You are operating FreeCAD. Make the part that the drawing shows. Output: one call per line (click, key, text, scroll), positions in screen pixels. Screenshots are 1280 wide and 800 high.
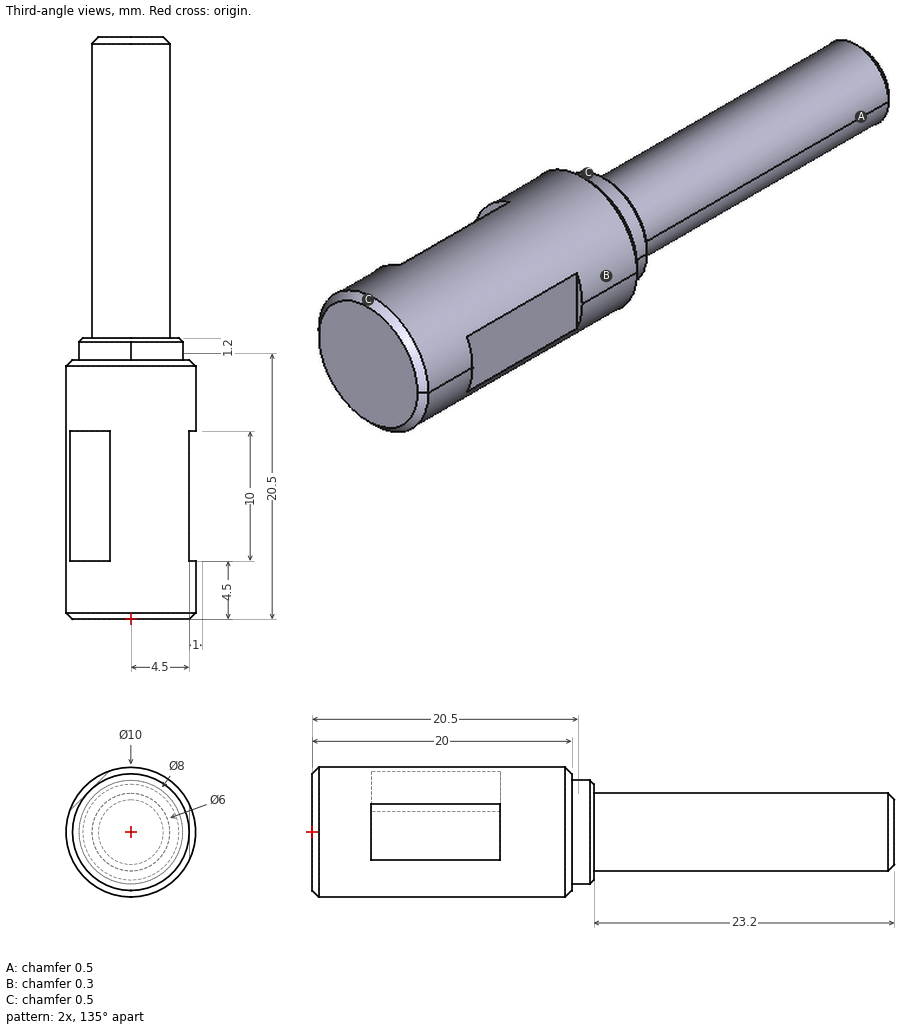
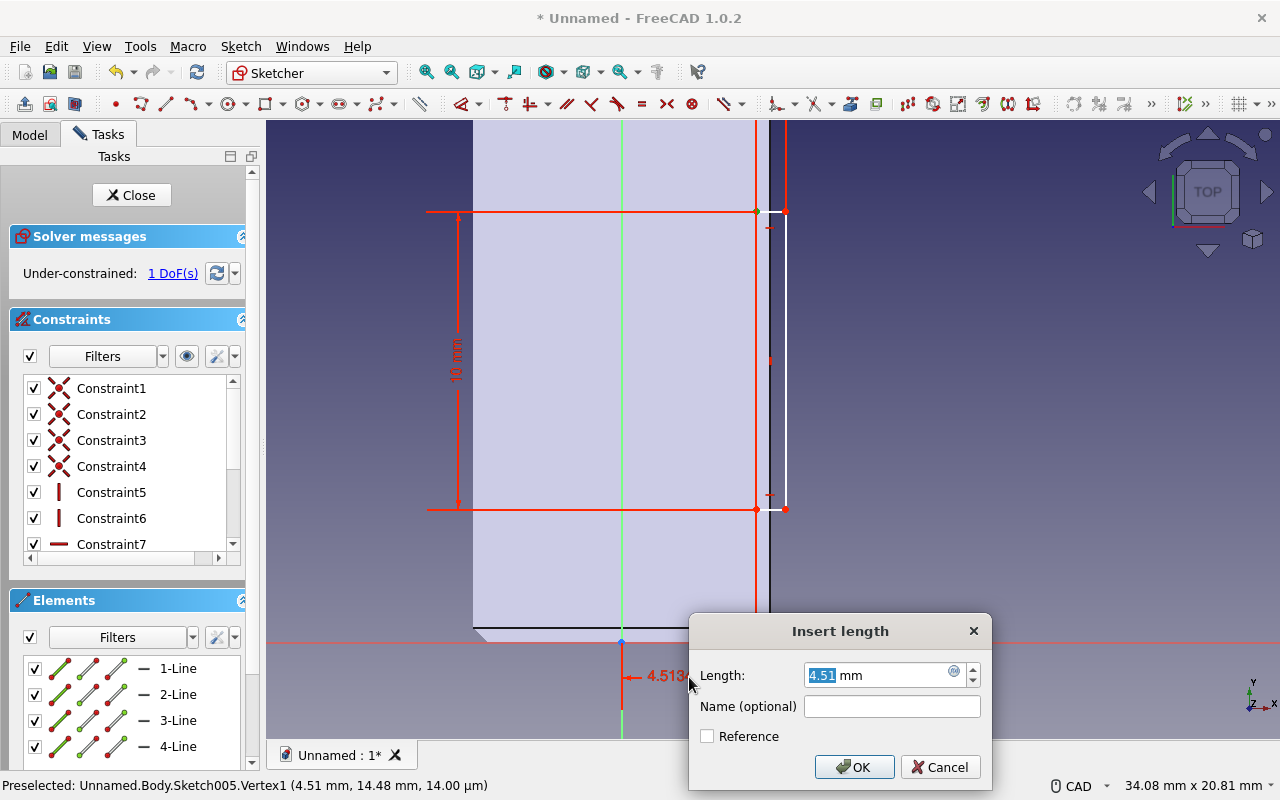
text(4.5)
key(Return)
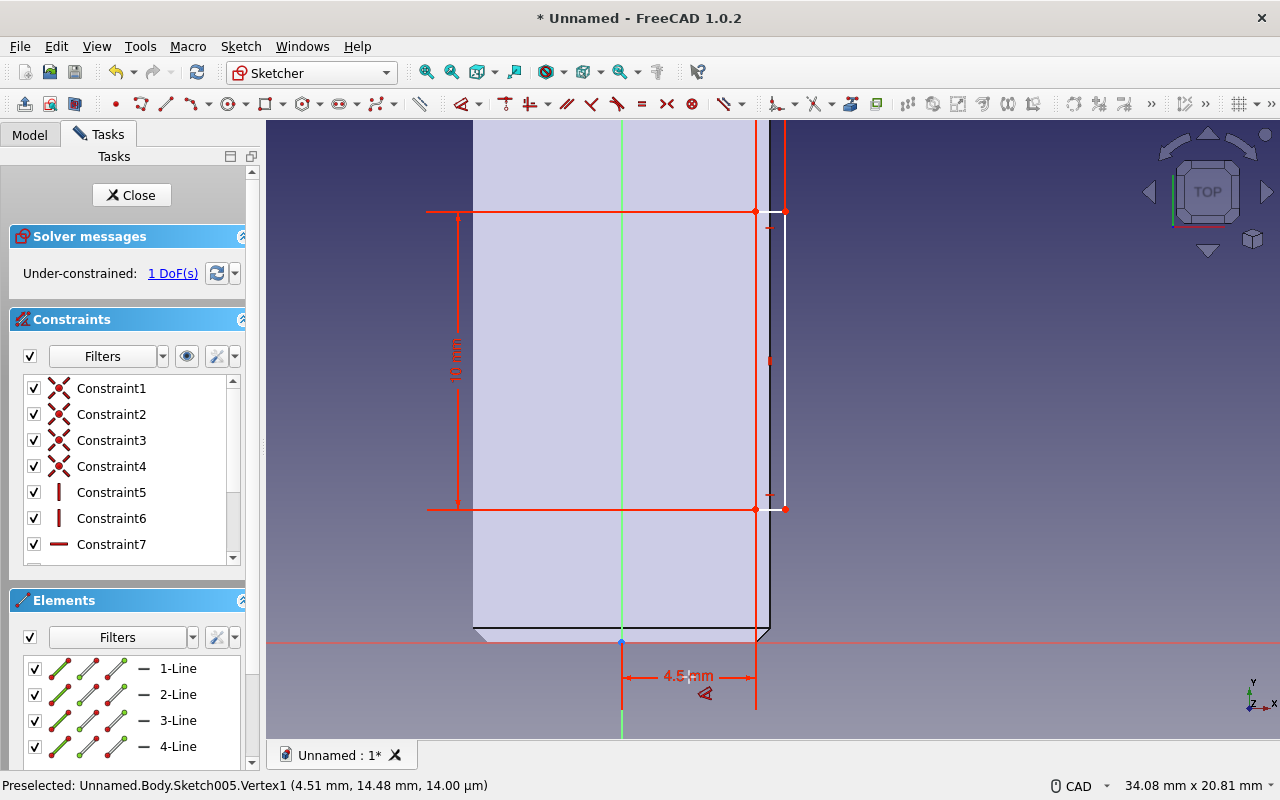
click(756, 510)
click(588, 576)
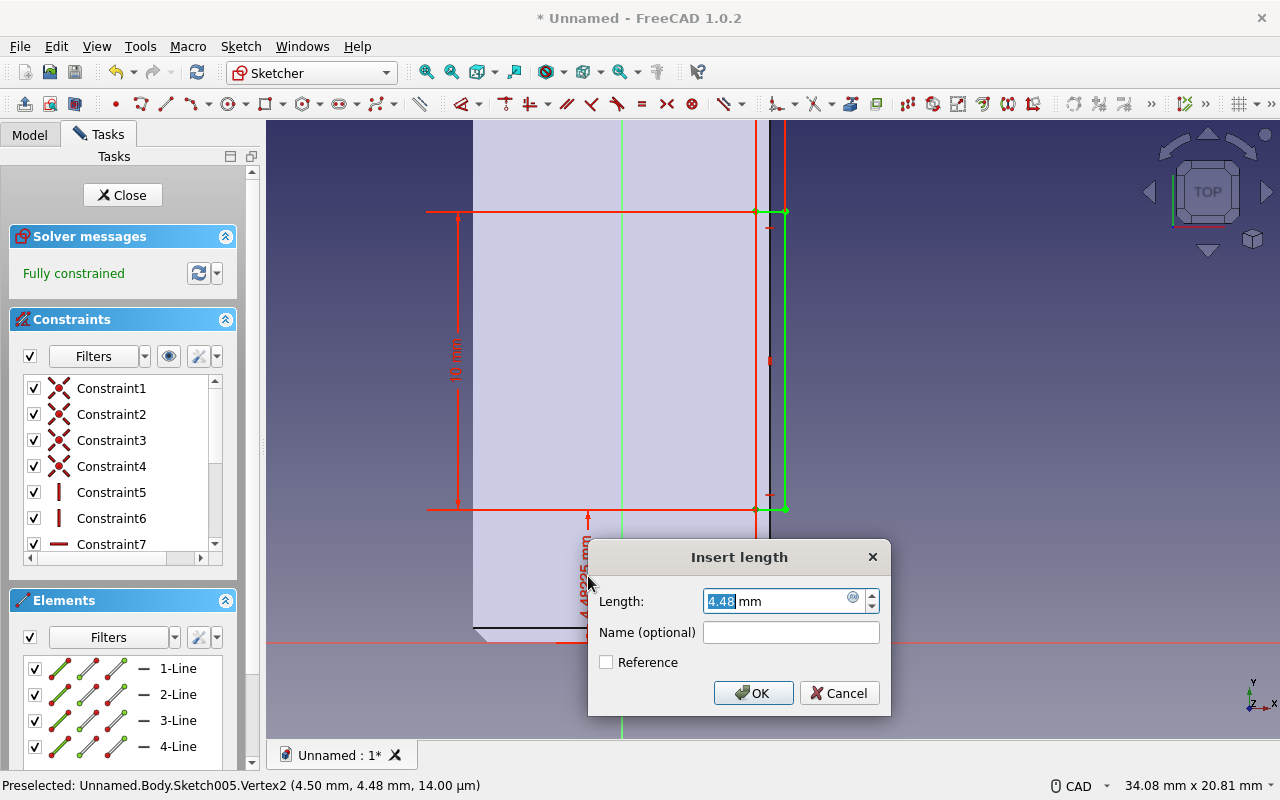
text(4.5)
key(Return)
key(Escape)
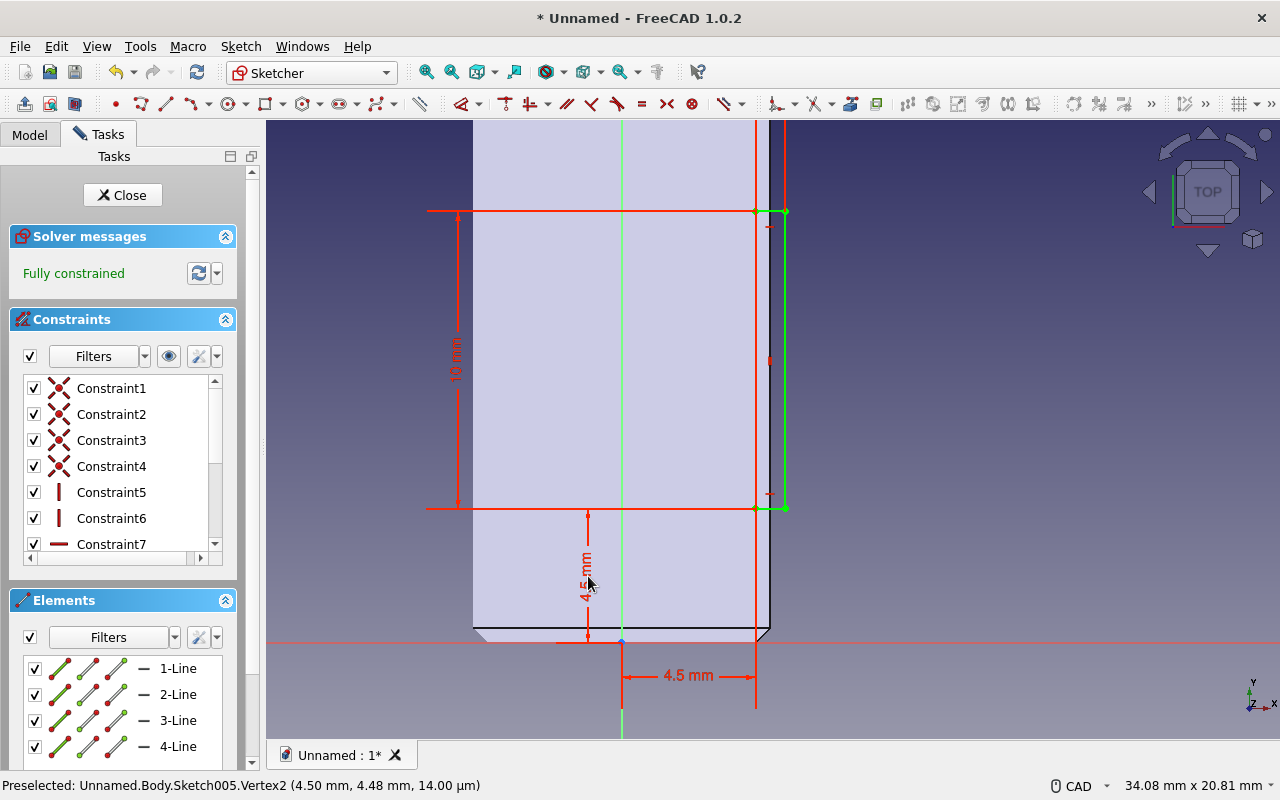
click(123, 195)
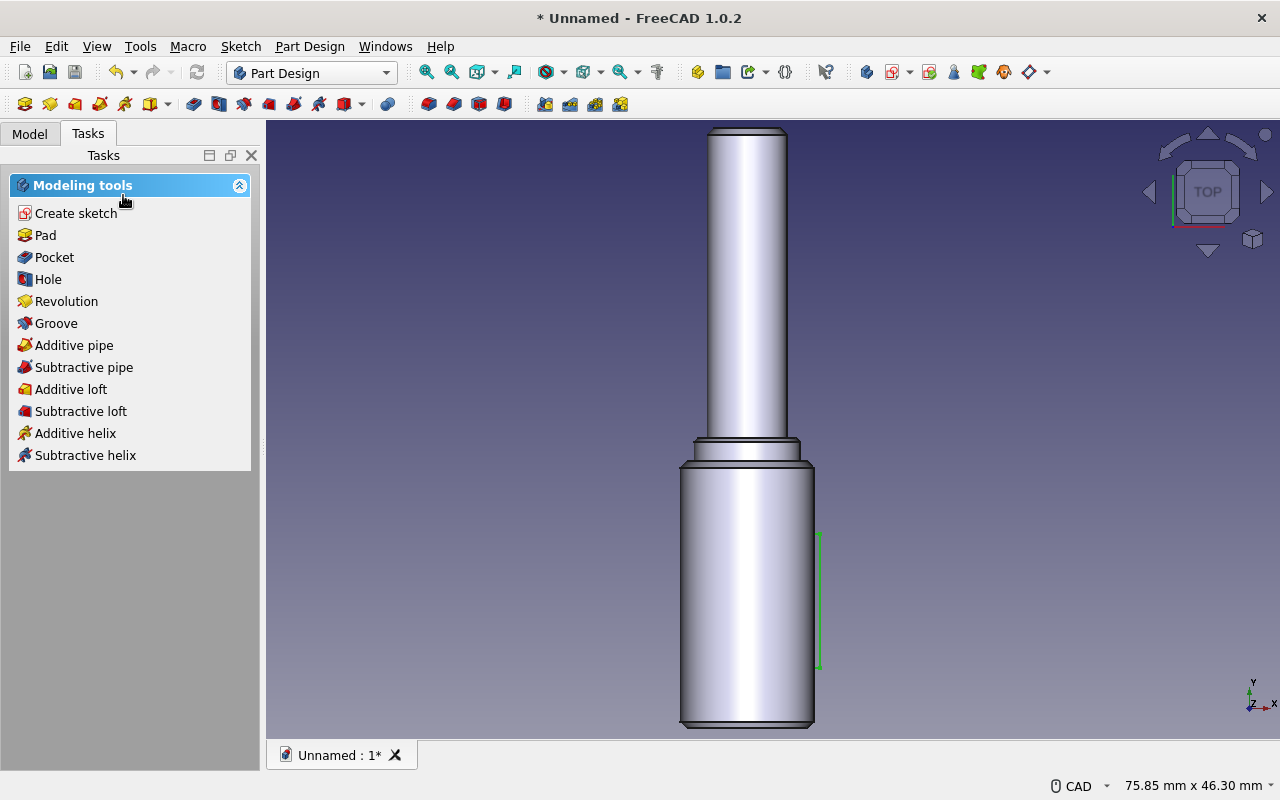
click(194, 104)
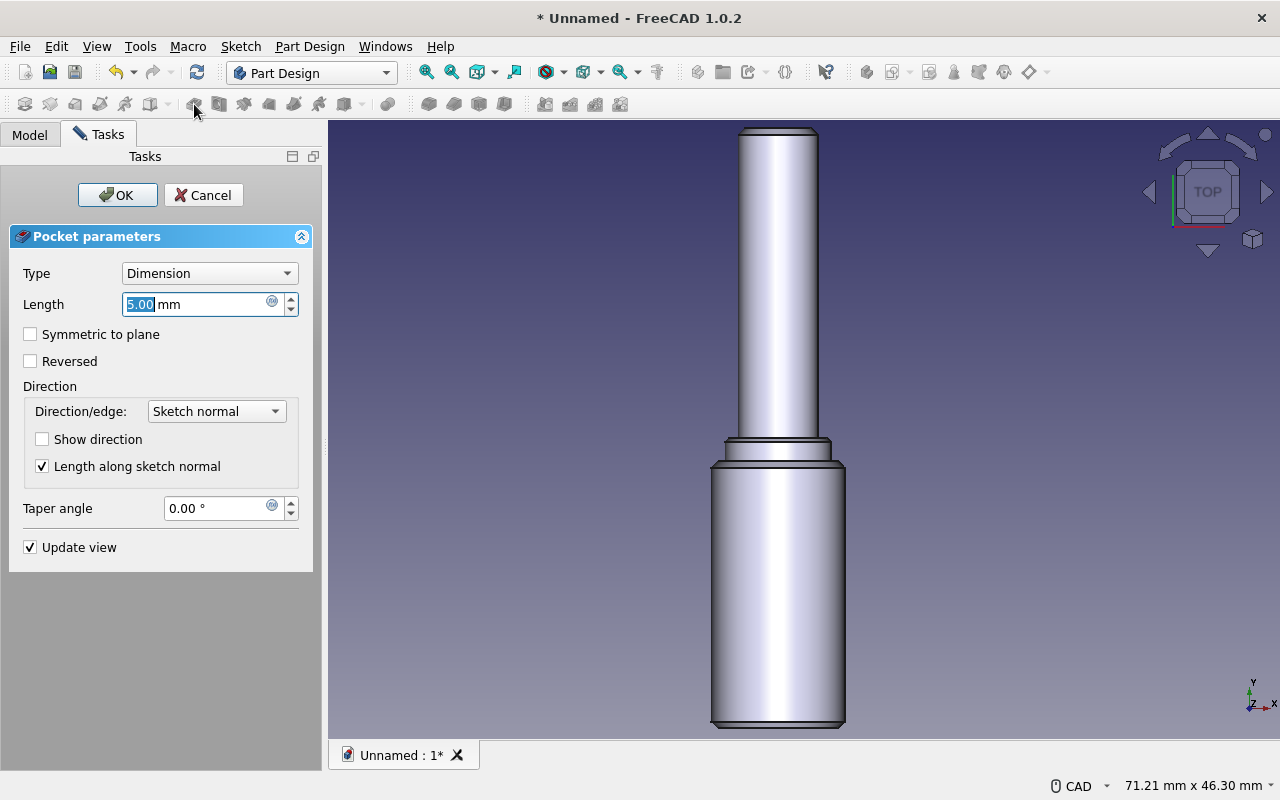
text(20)
key(Tab)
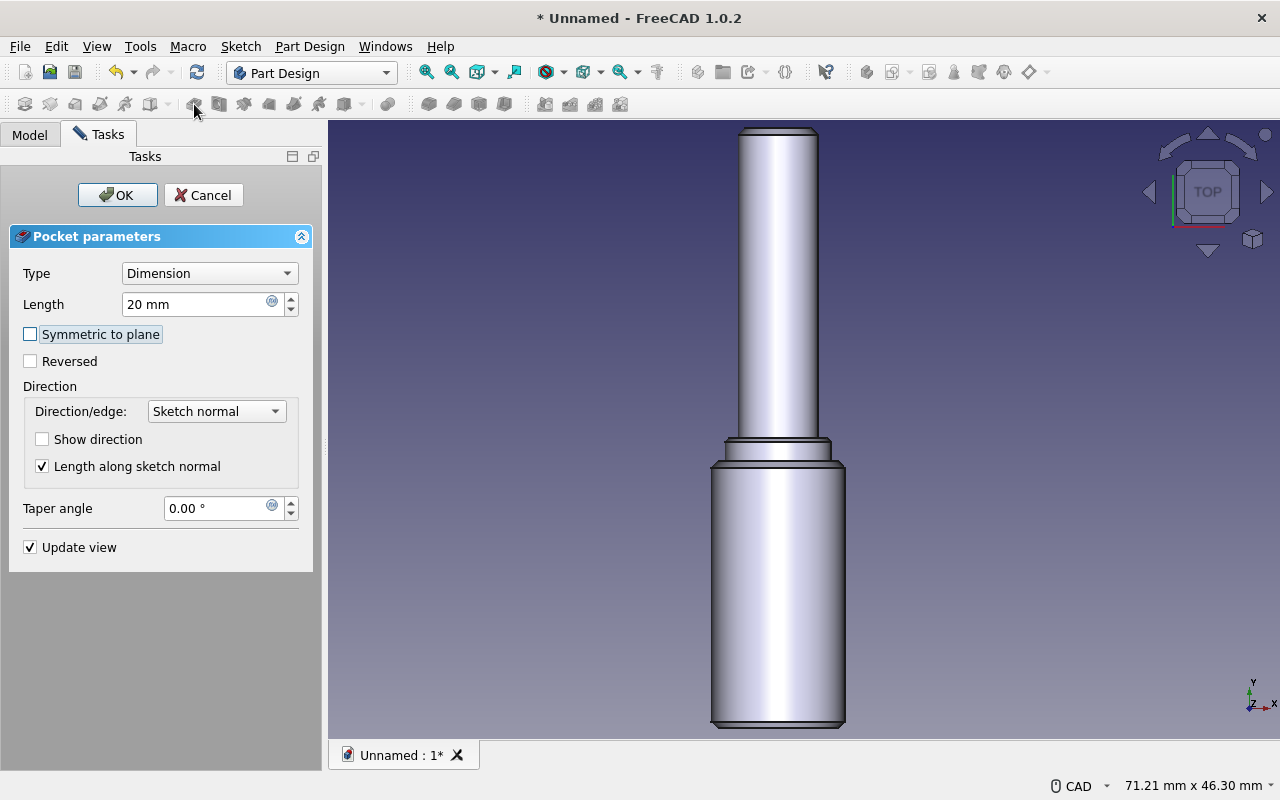
click(31, 334)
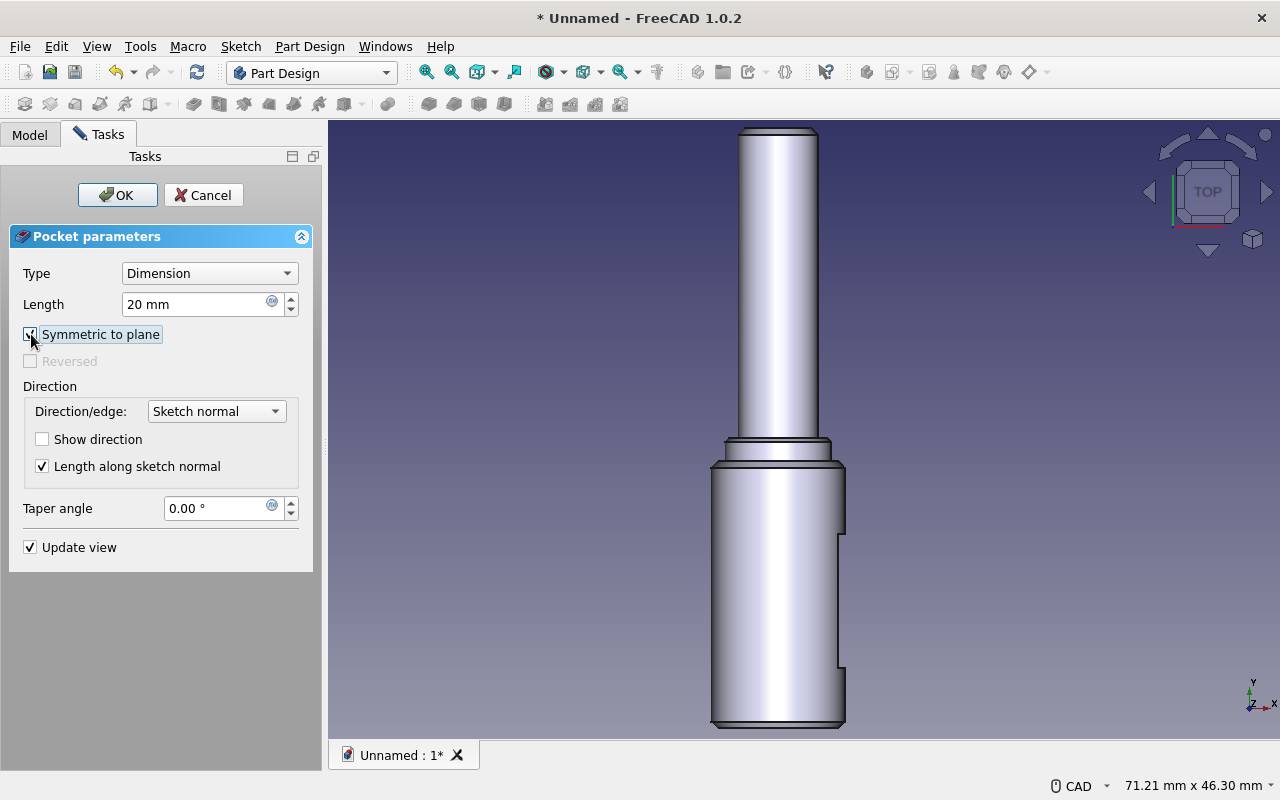
click(118, 195)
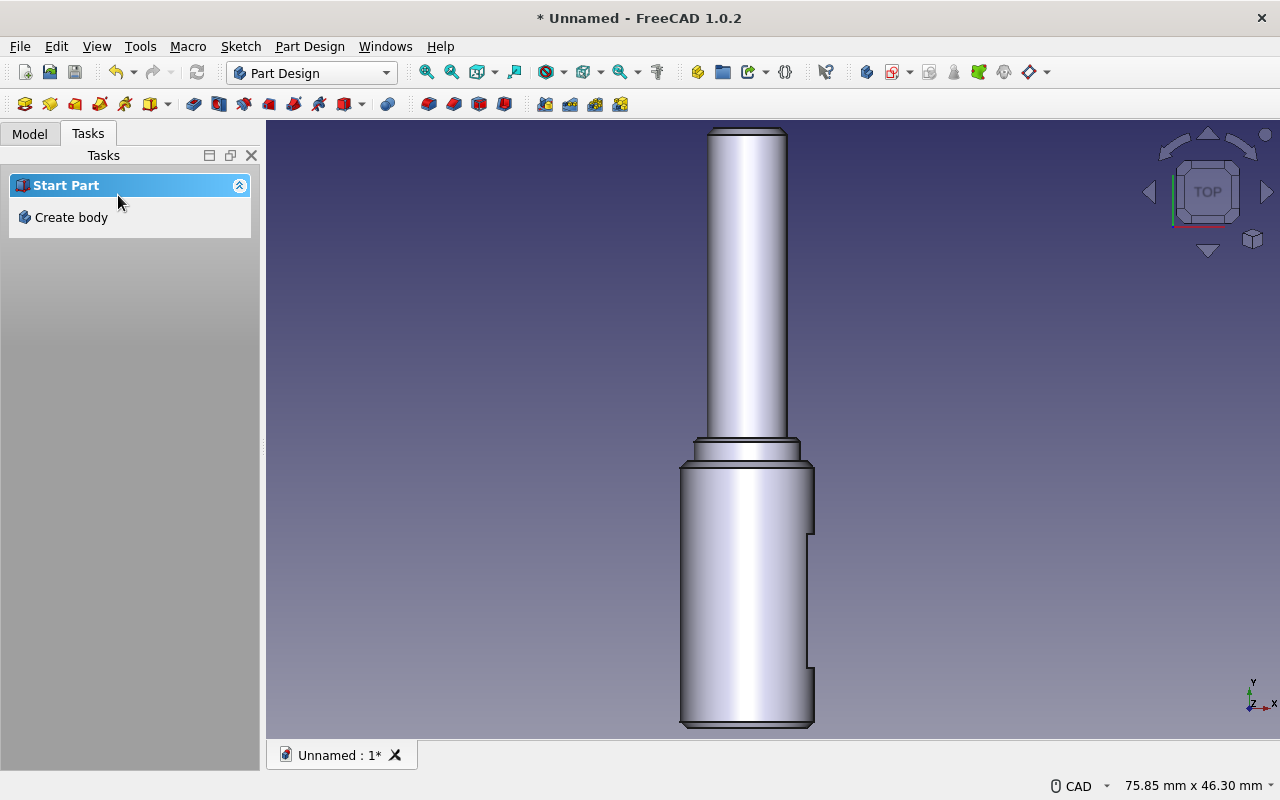
click(30, 134)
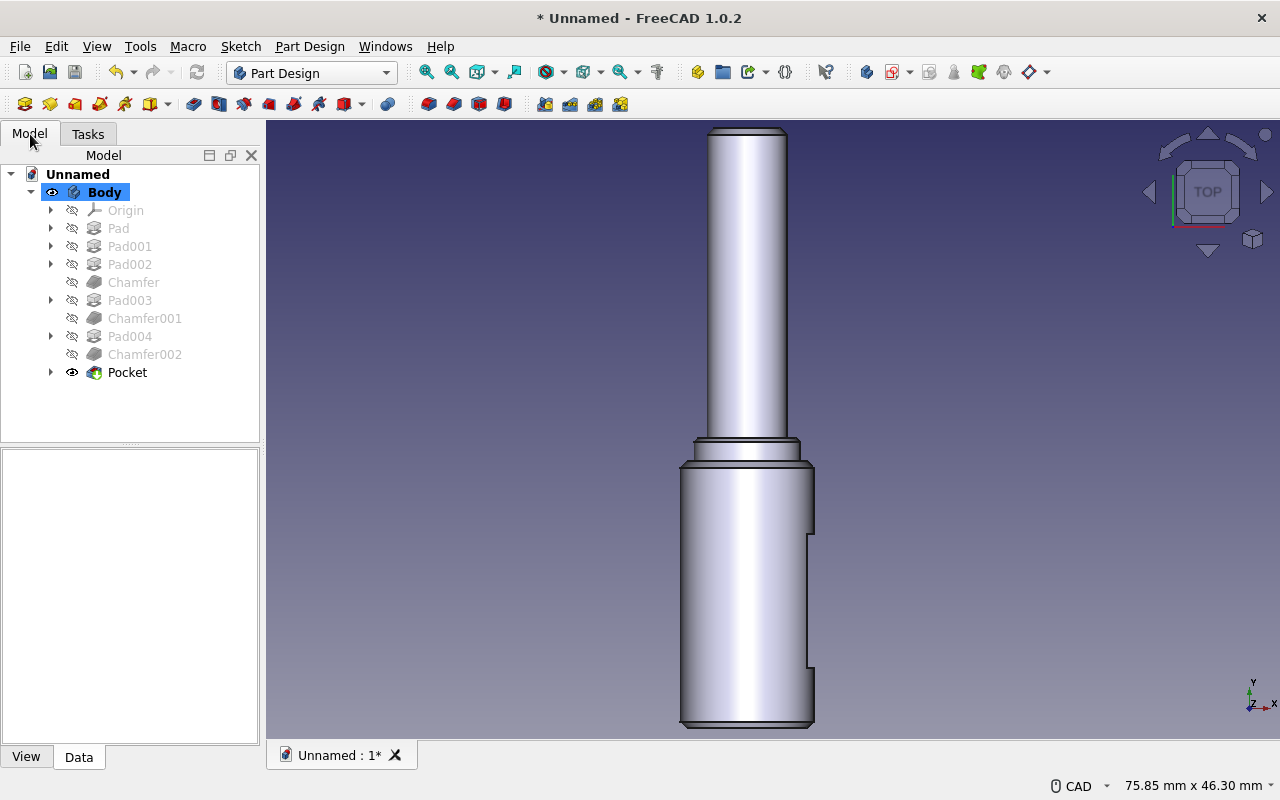
click(117, 372)